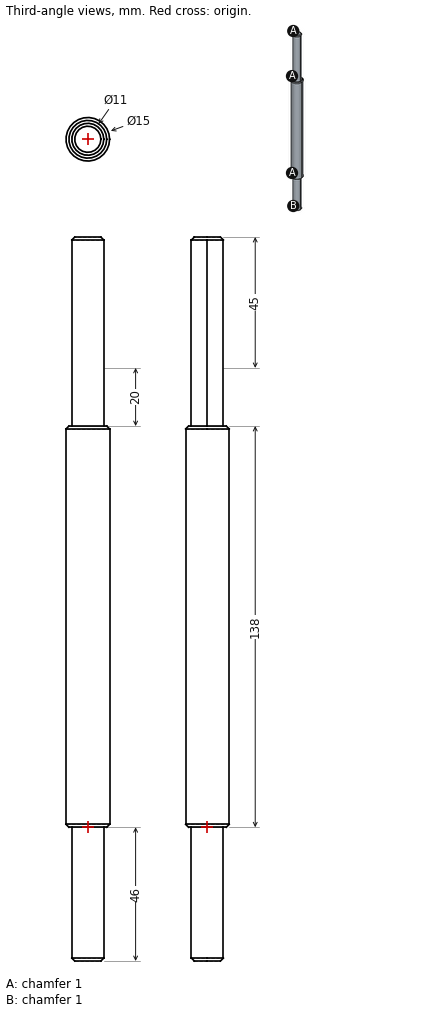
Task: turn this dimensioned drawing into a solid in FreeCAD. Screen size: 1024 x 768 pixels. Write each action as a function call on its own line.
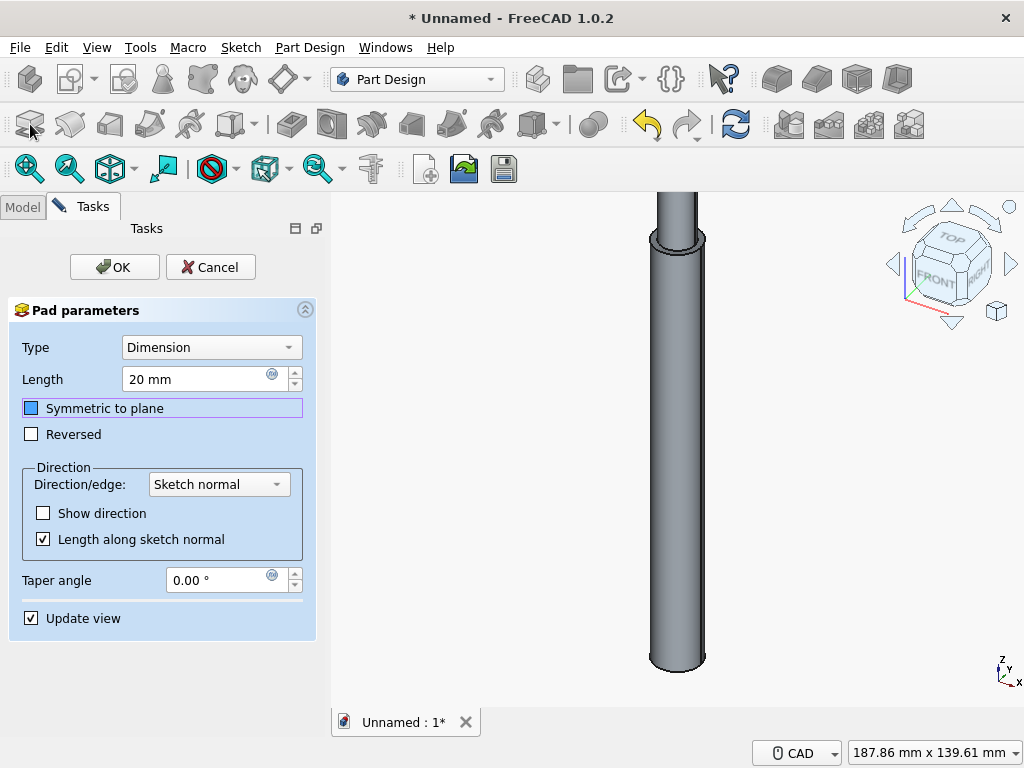
click(115, 267)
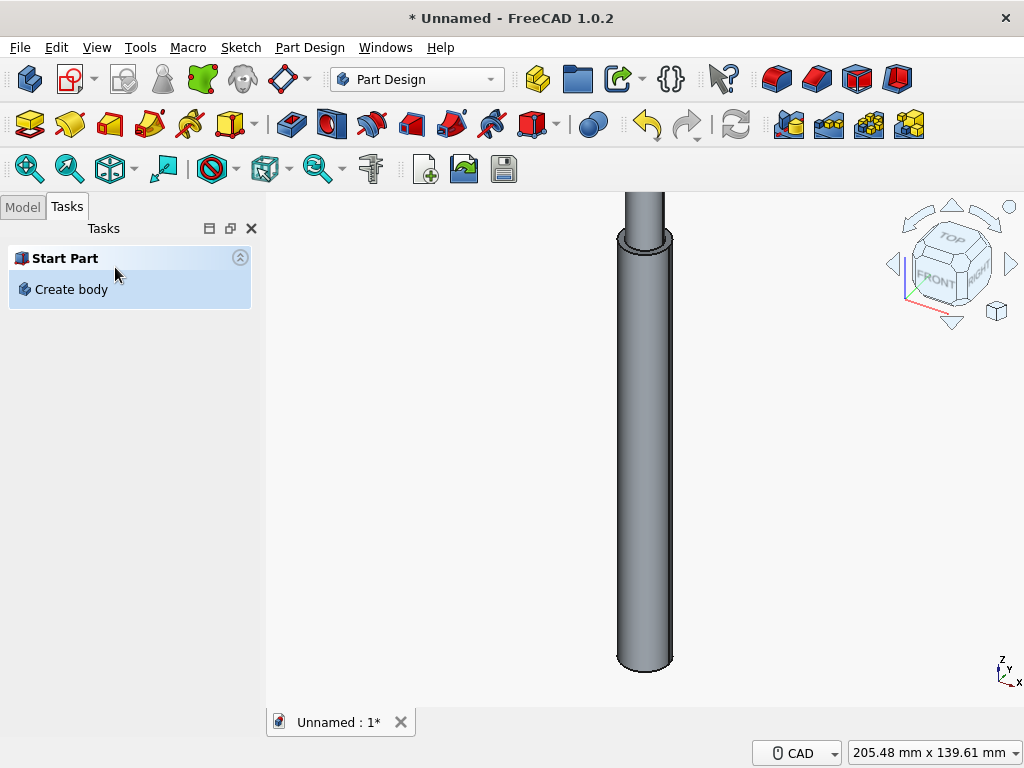
click(30, 170)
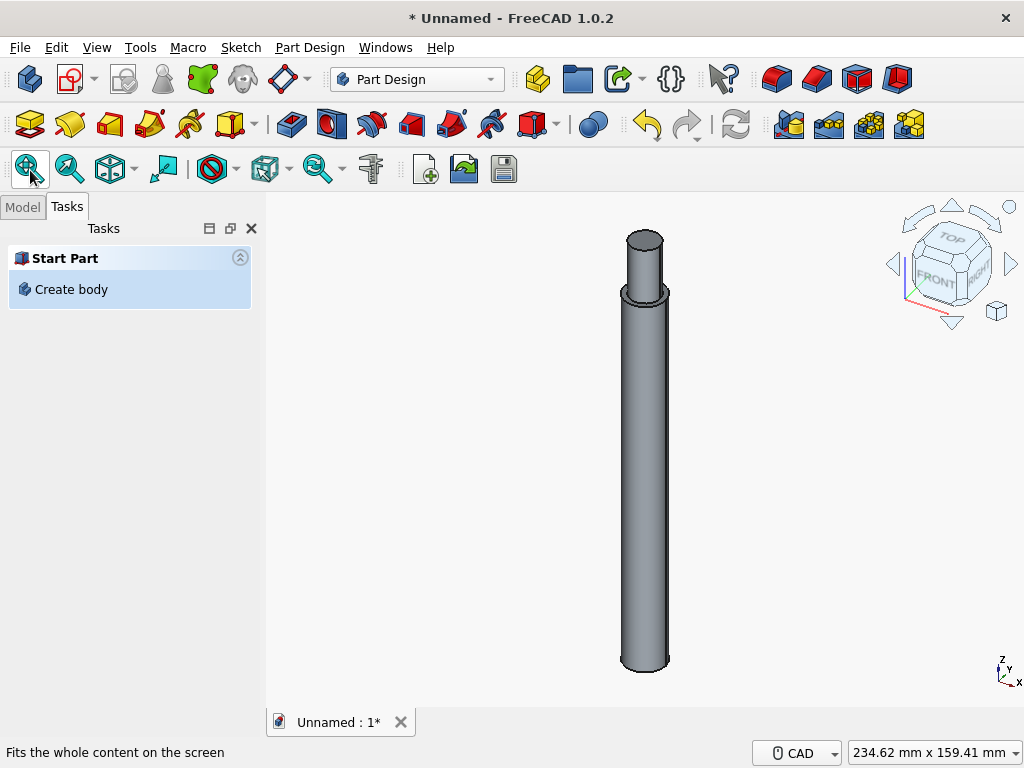
click(645, 239)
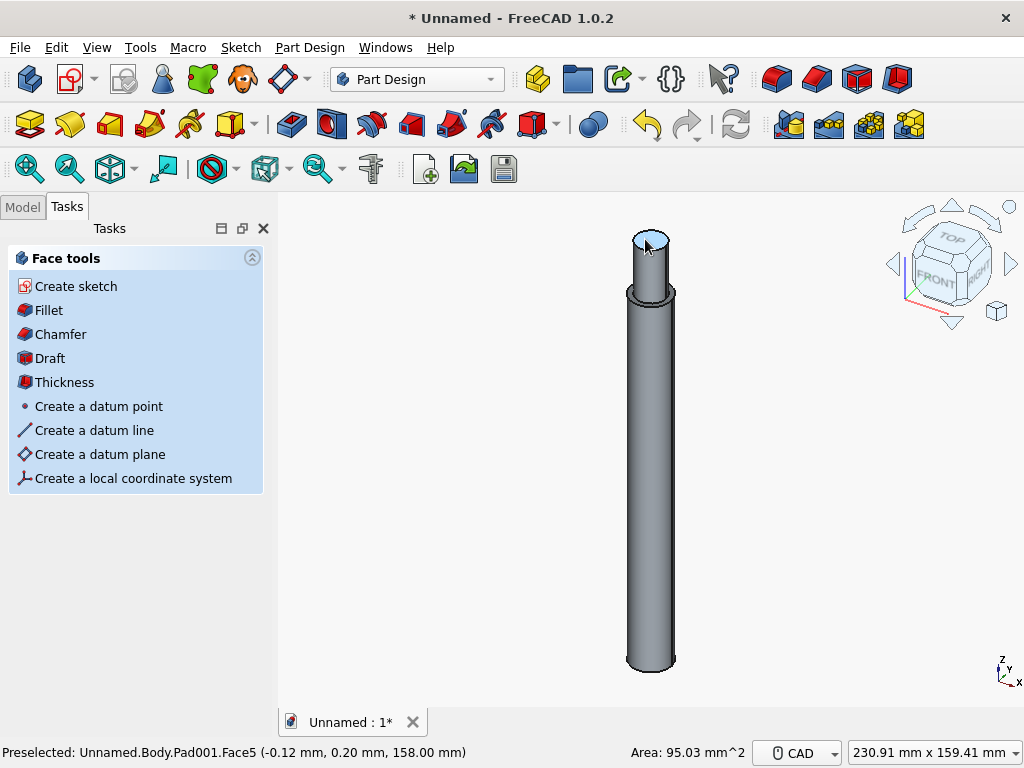
click(70, 80)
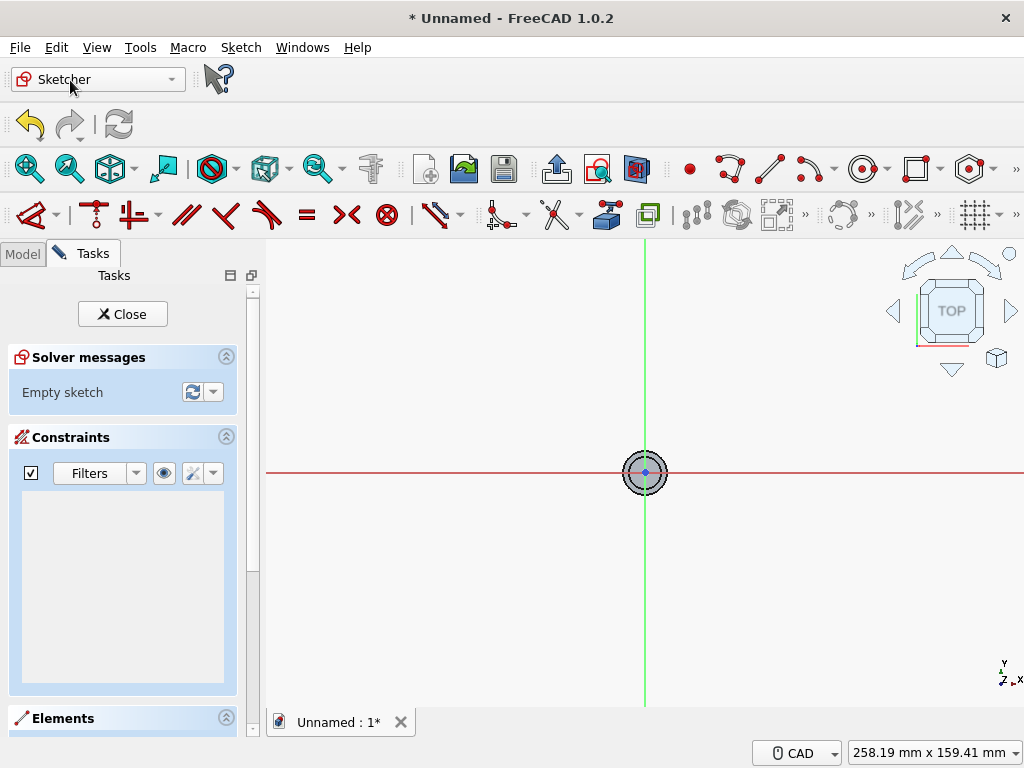
scroll(654, 473, up, 11)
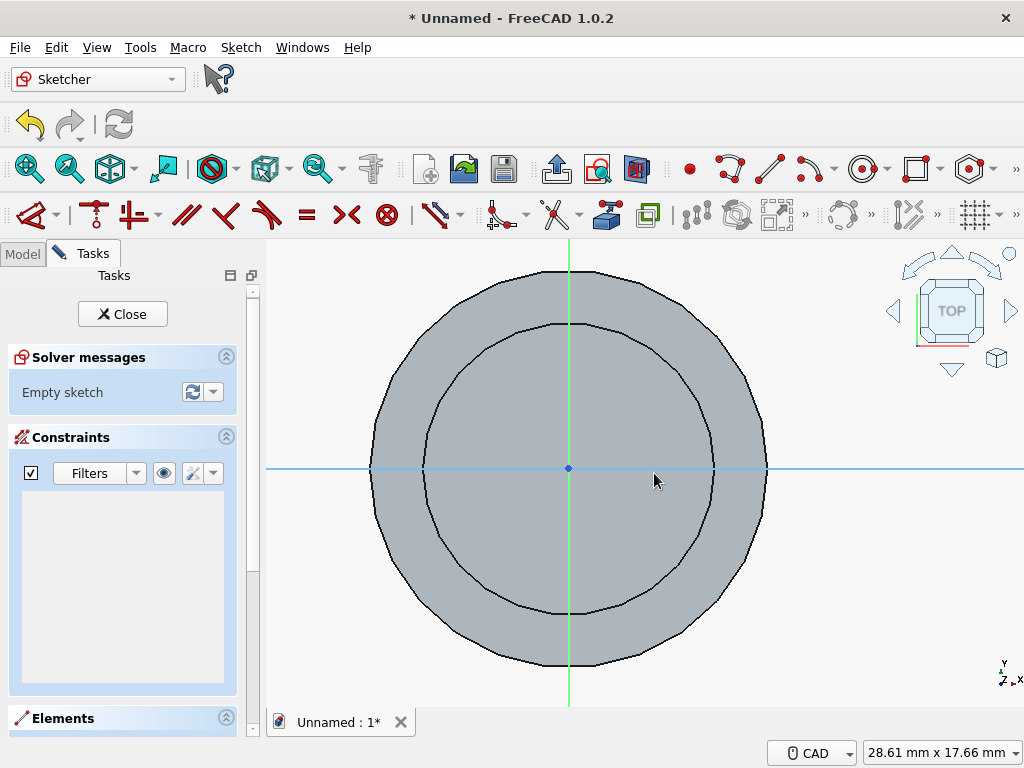
click(864, 170)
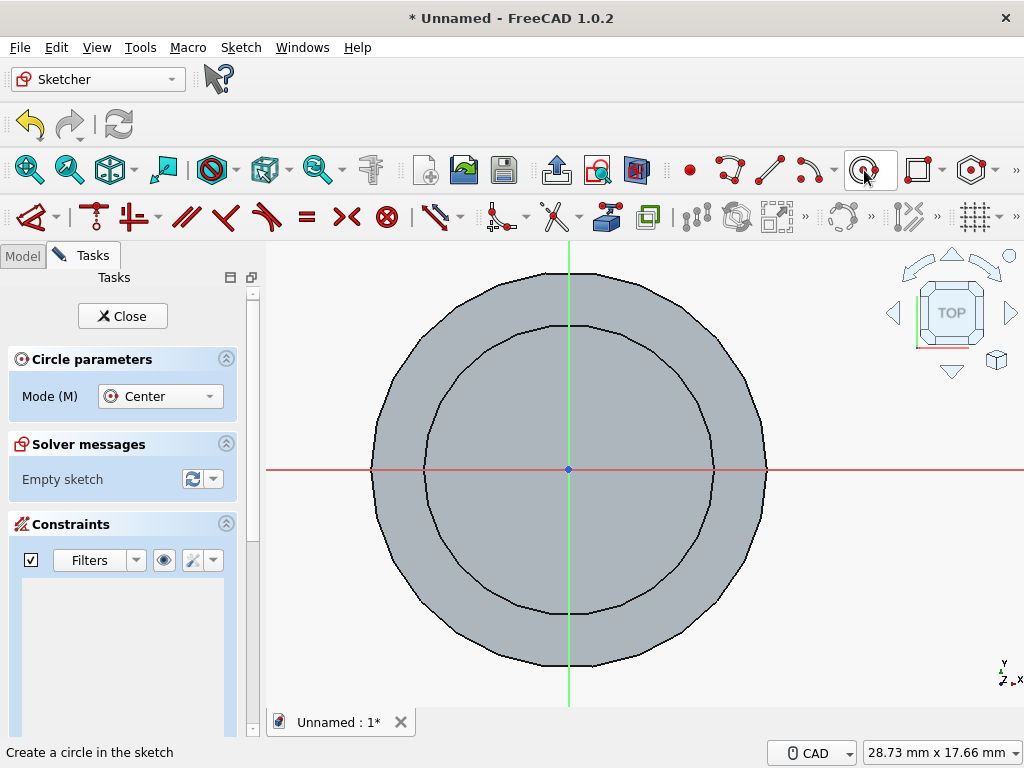
click(569, 470)
click(672, 367)
key(Escape)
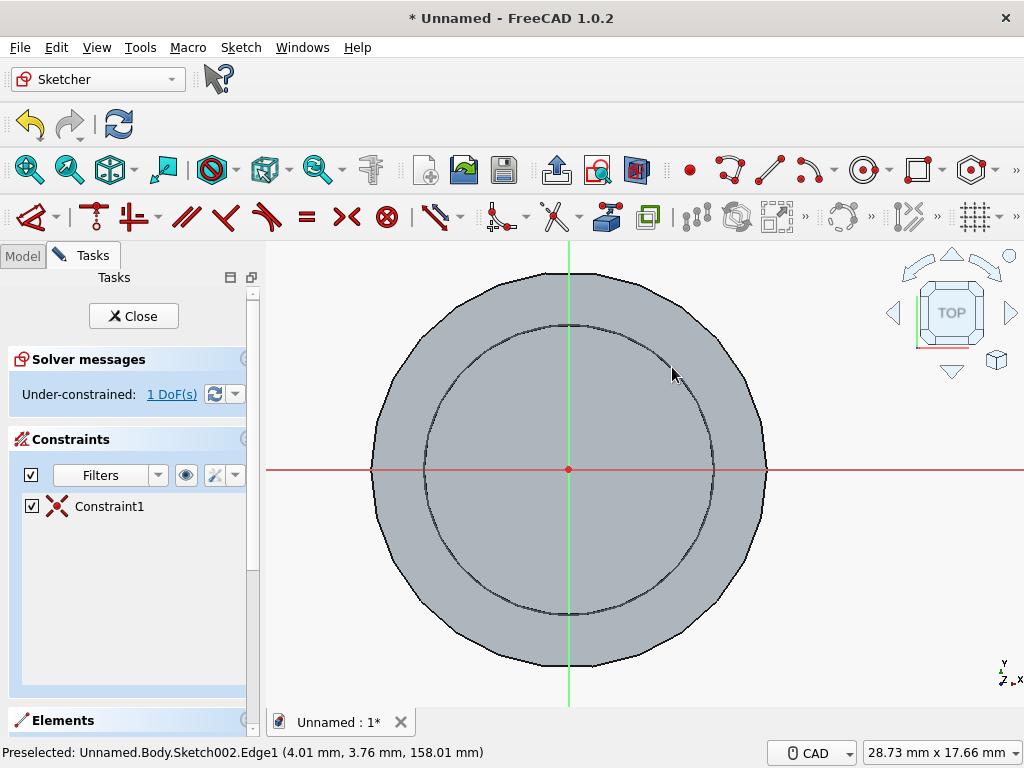
click(32, 218)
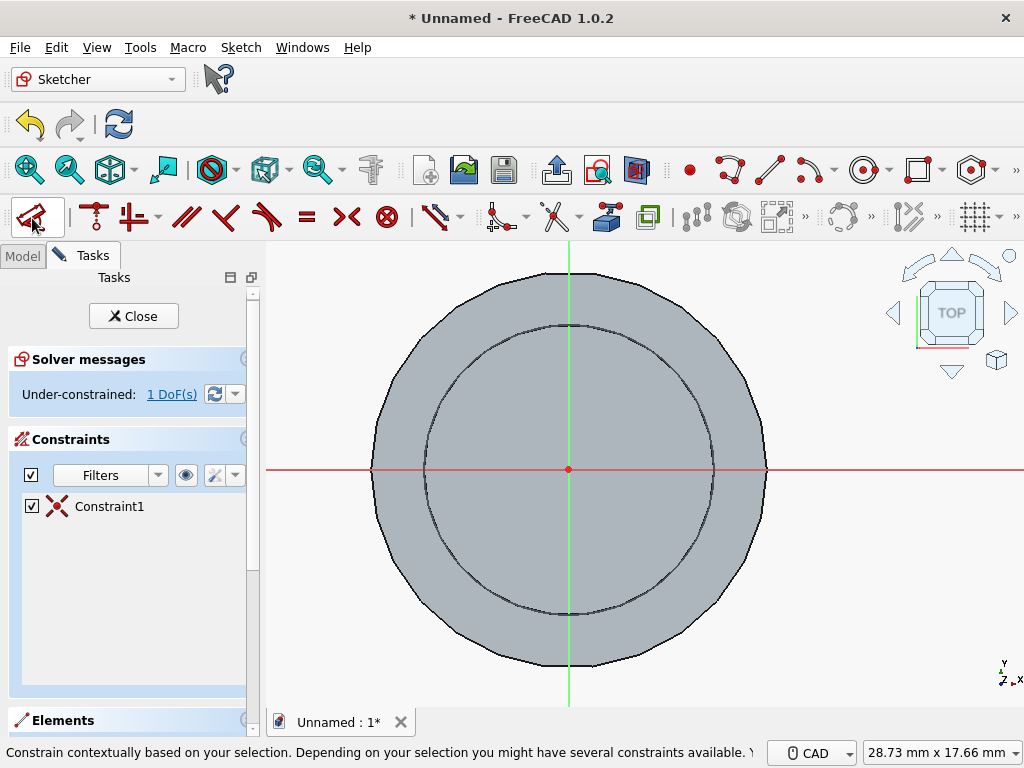
click(671, 367)
click(694, 344)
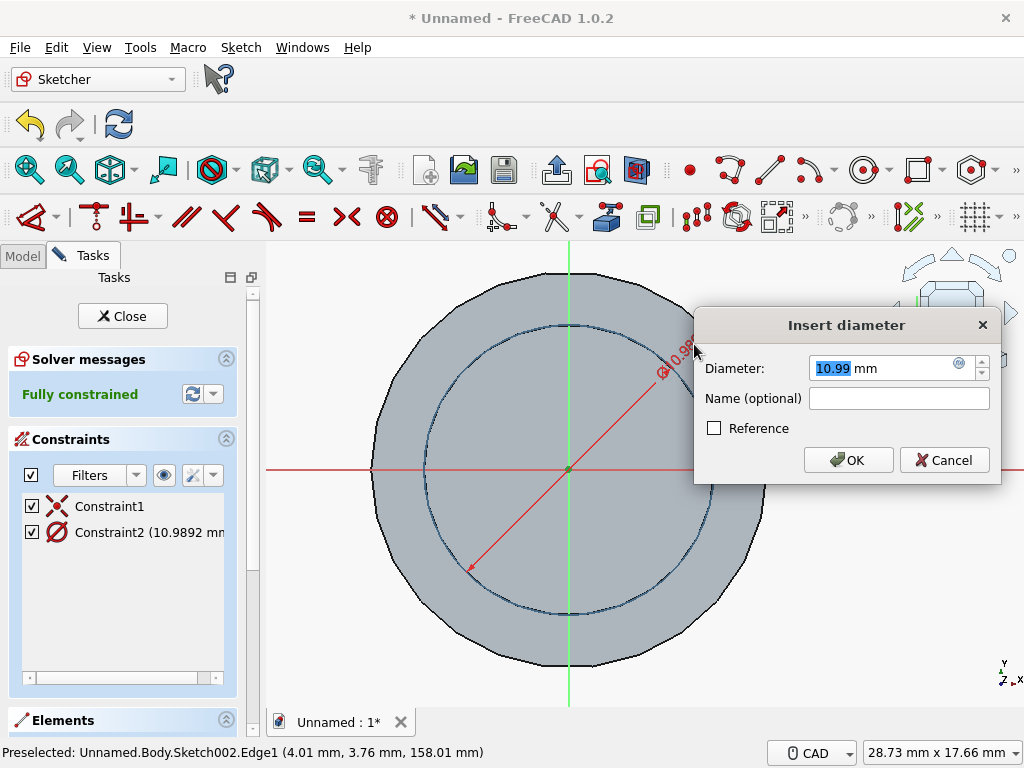
text(11)
key(Return)
key(Escape)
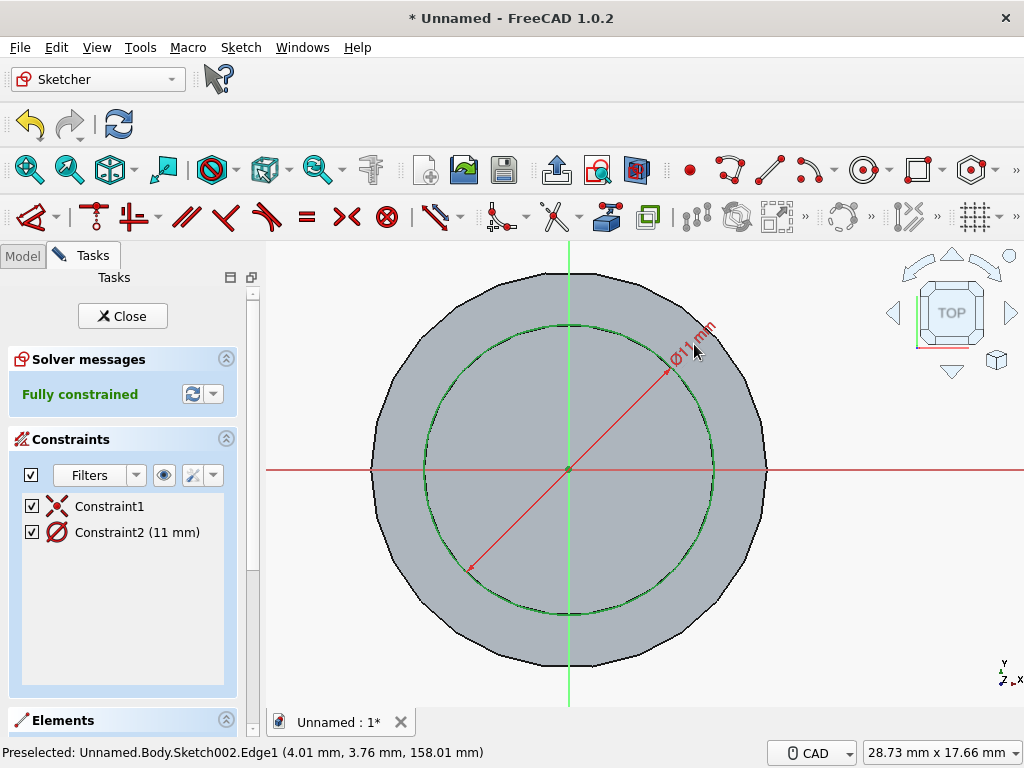
click(123, 316)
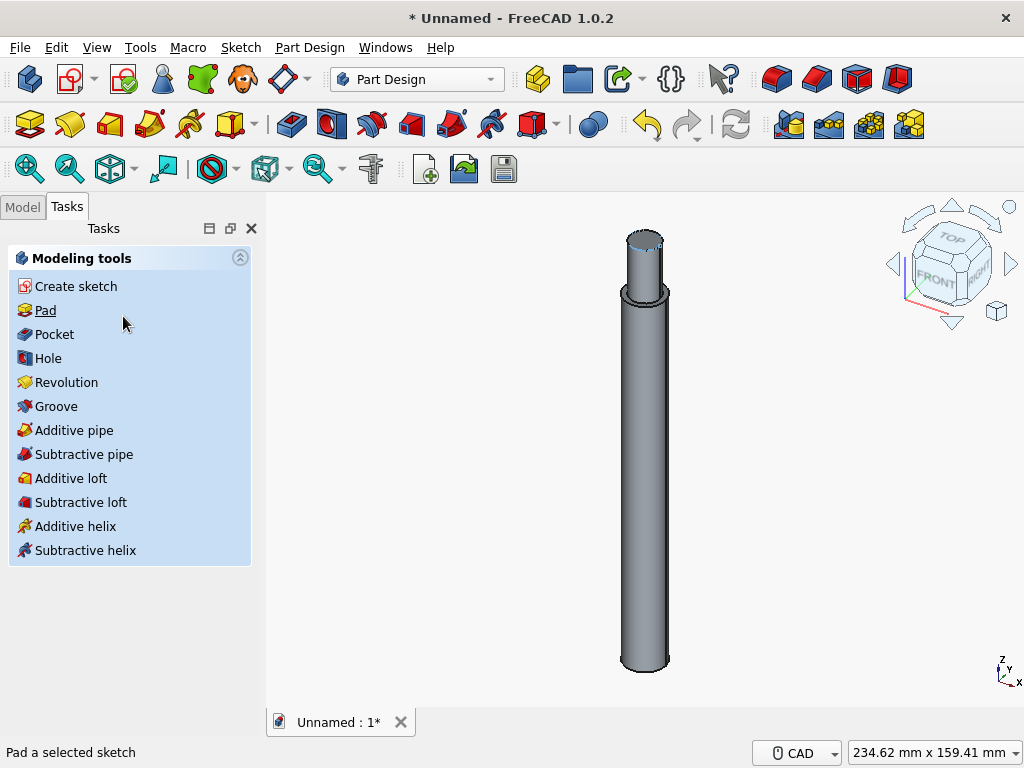
click(30, 124)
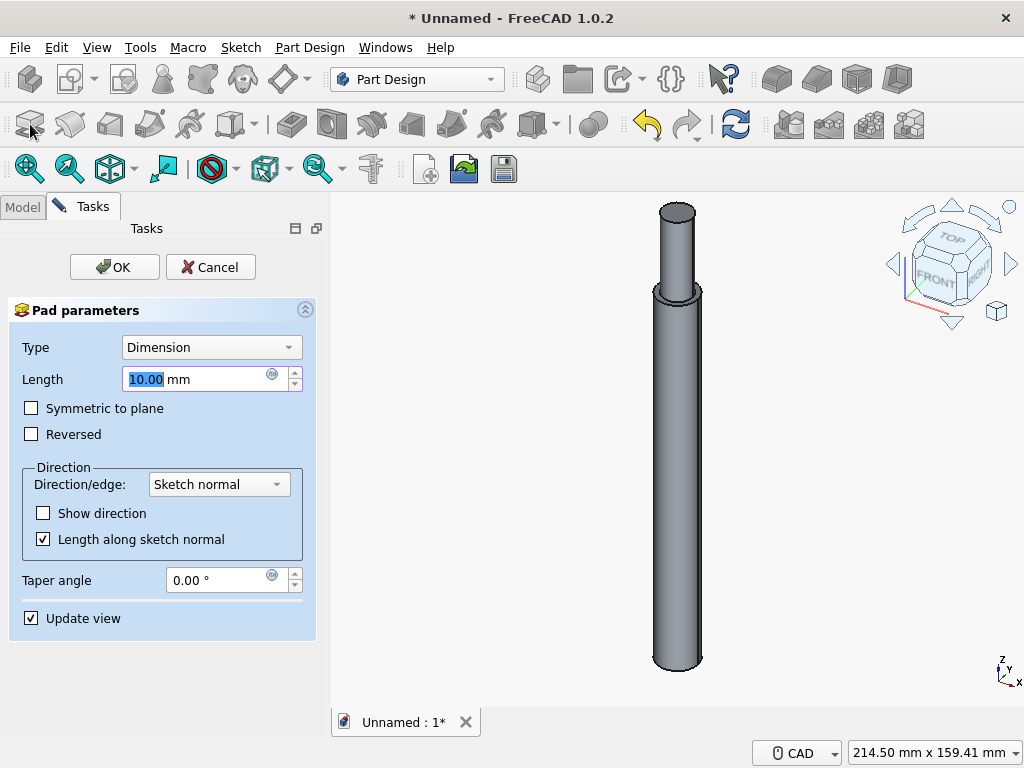
text(45)
key(Tab)